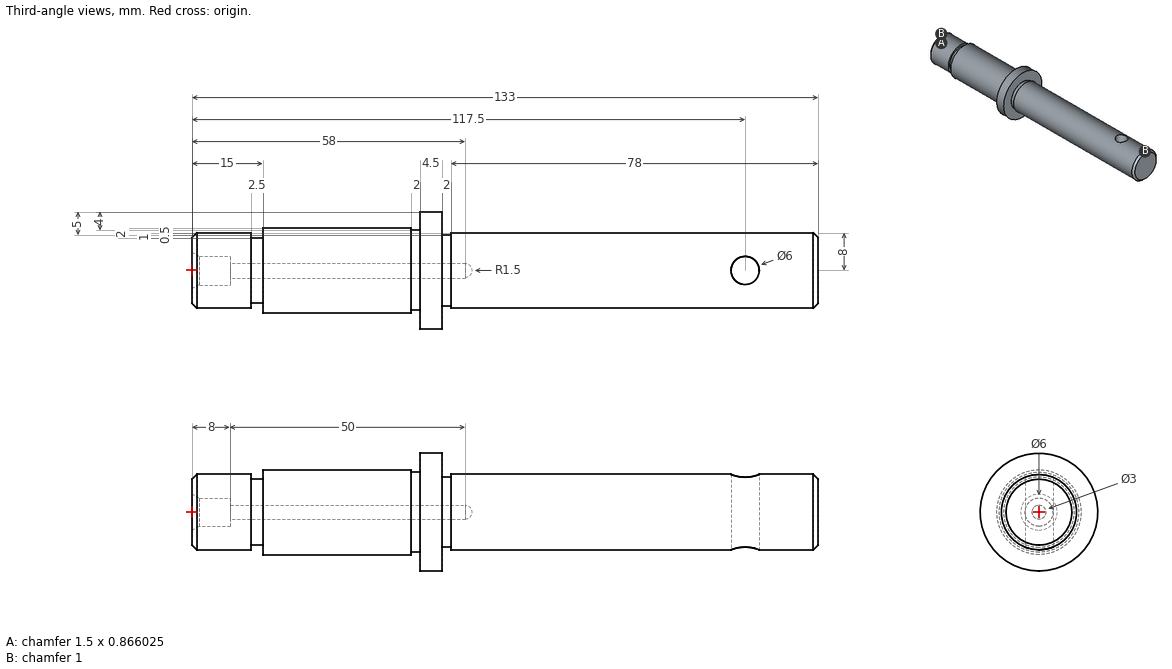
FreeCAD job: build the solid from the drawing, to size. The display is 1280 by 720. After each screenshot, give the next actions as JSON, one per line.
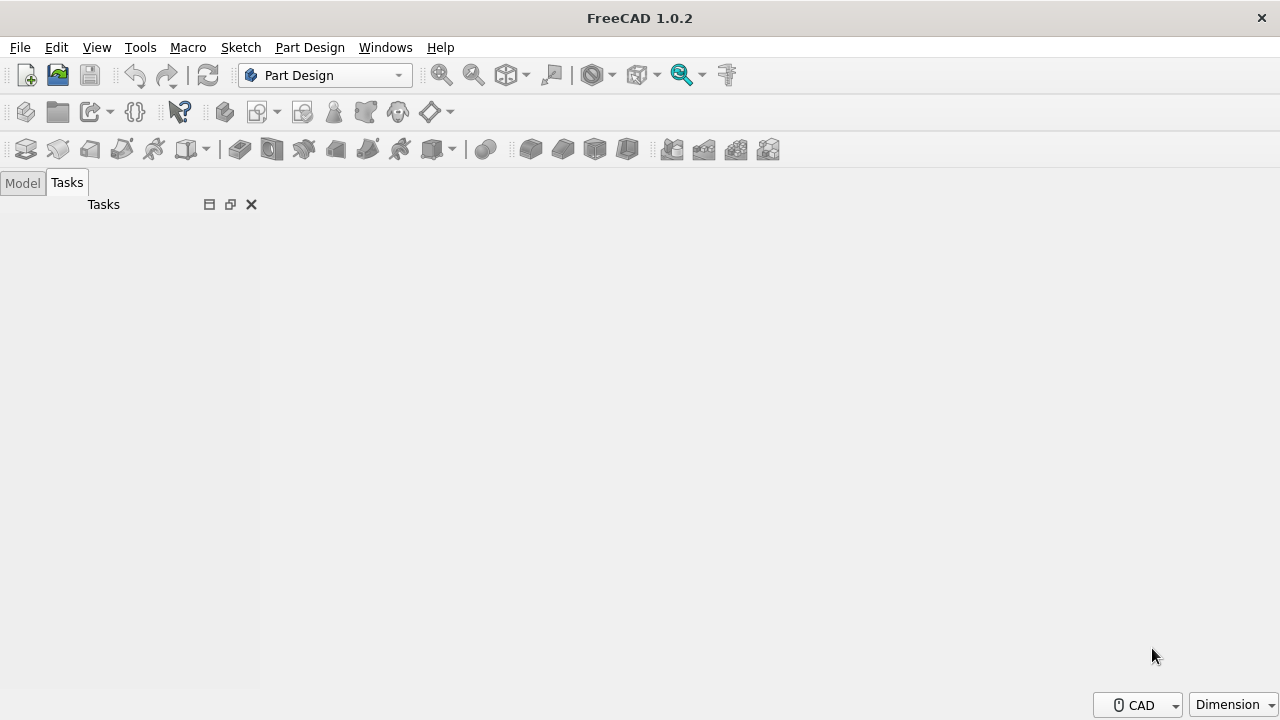
{"action": "left_click", "coordinate": [26, 76]}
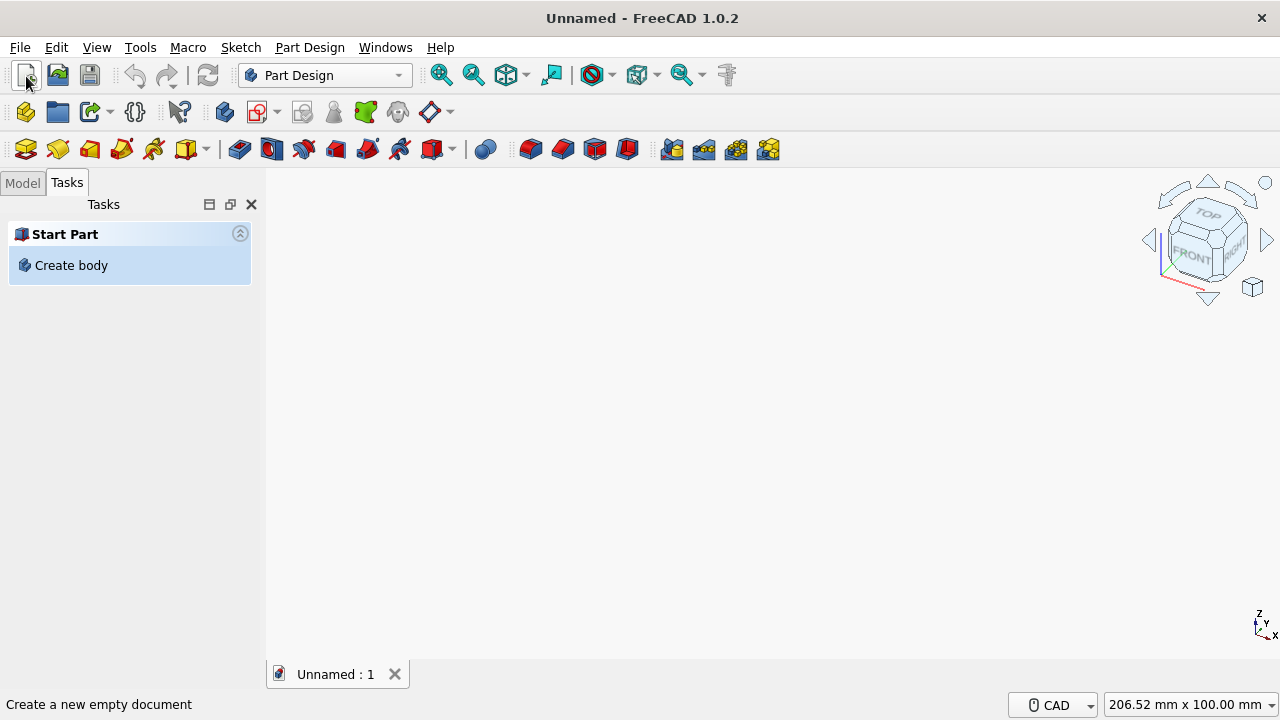
{"action": "left_click", "coordinate": [258, 112]}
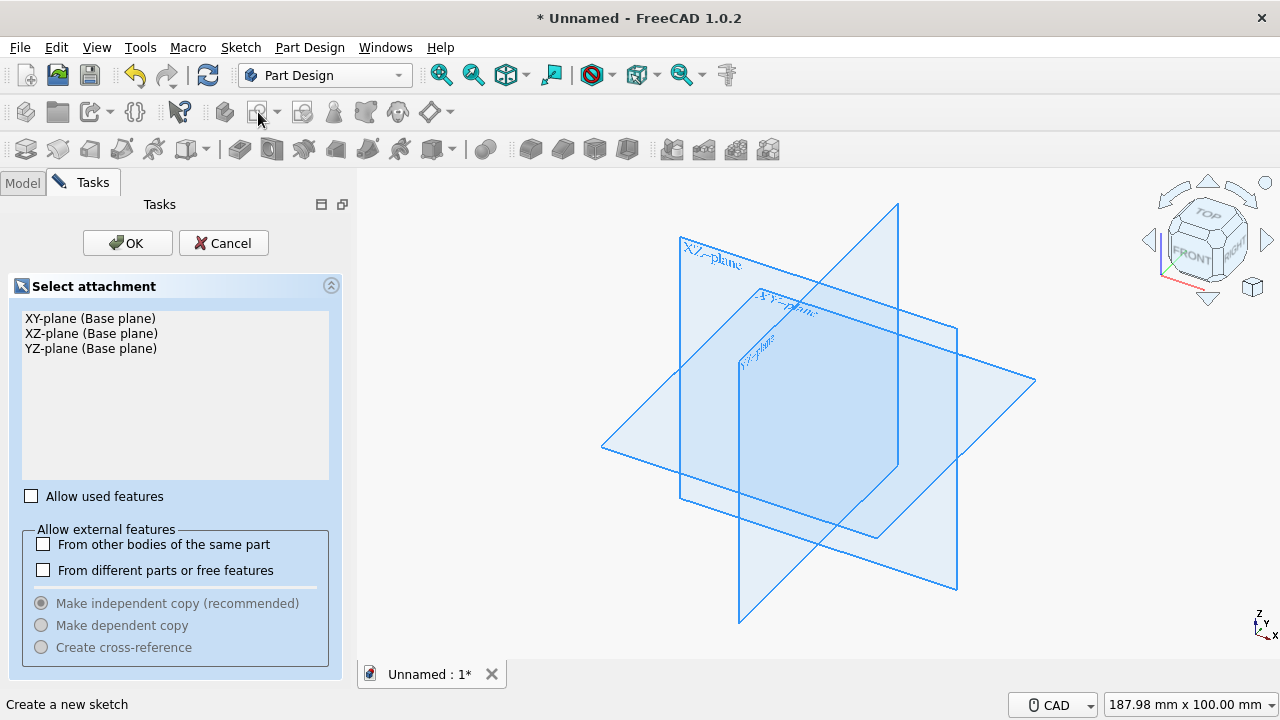
{"action": "left_click", "coordinate": [82, 318]}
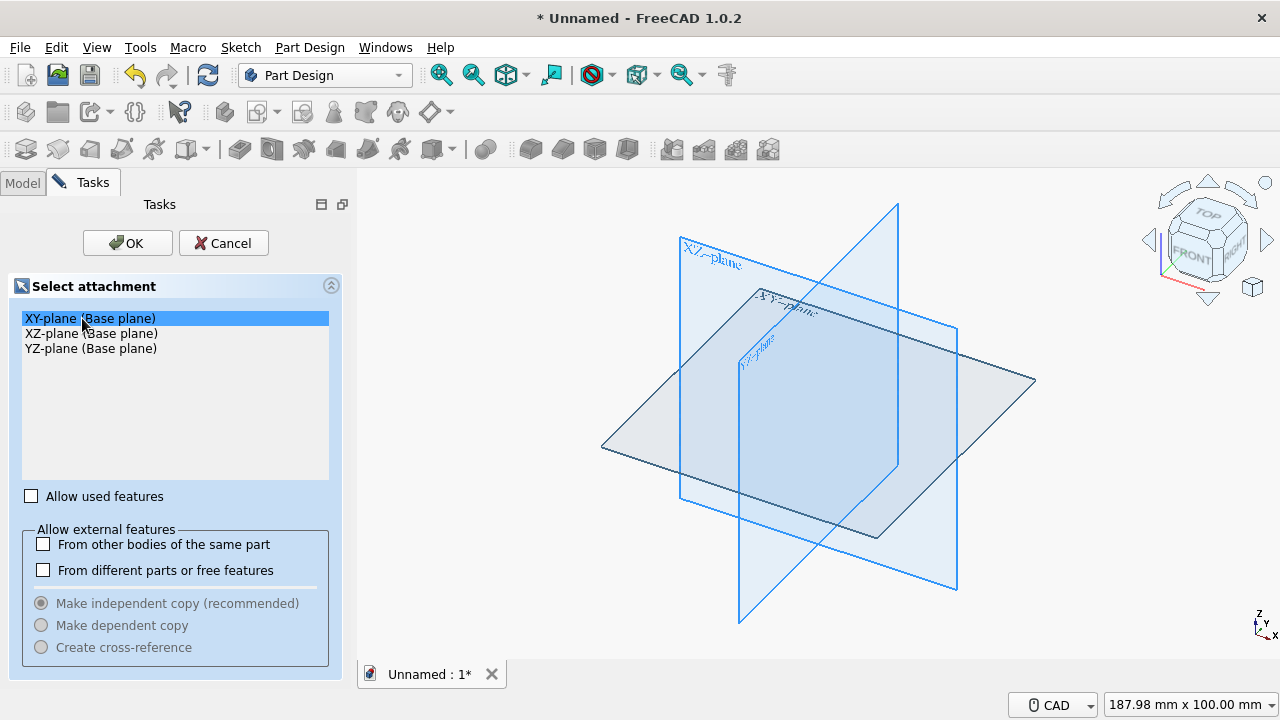
{"action": "left_click", "coordinate": [128, 243]}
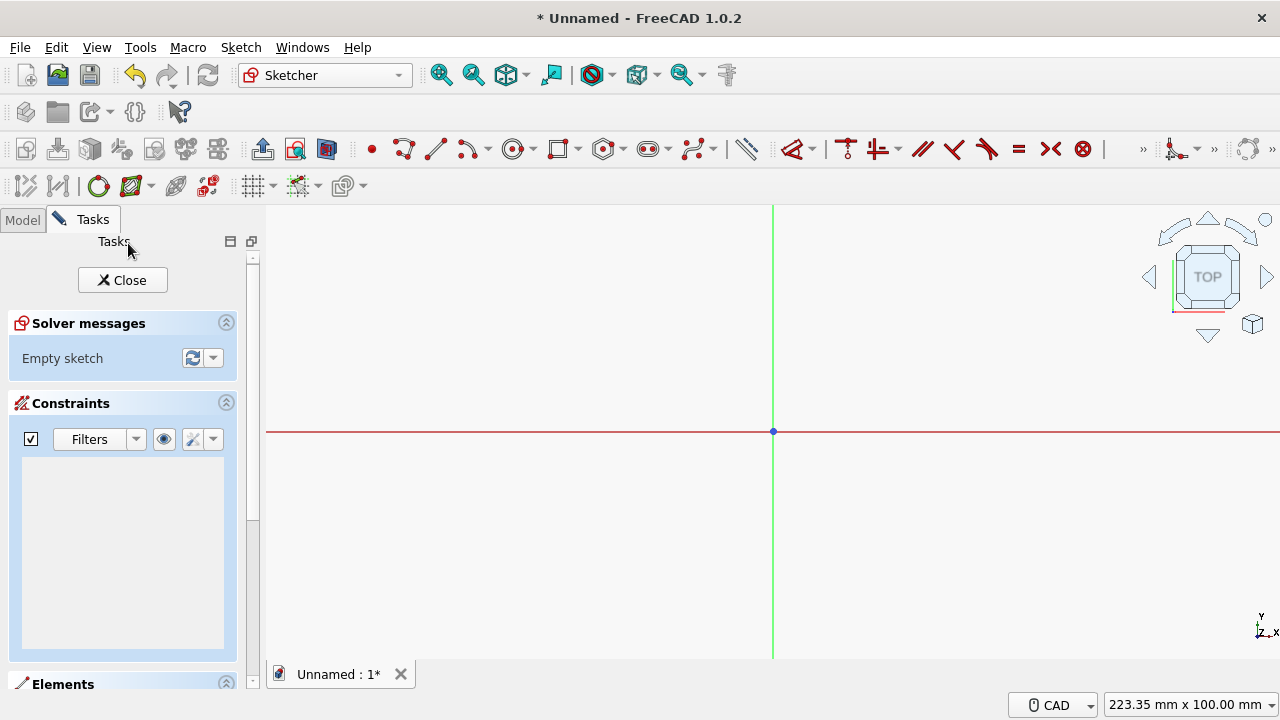
{"action": "scroll", "coordinate": [294, 490], "scroll_direction": "down", "scroll_amount": 2}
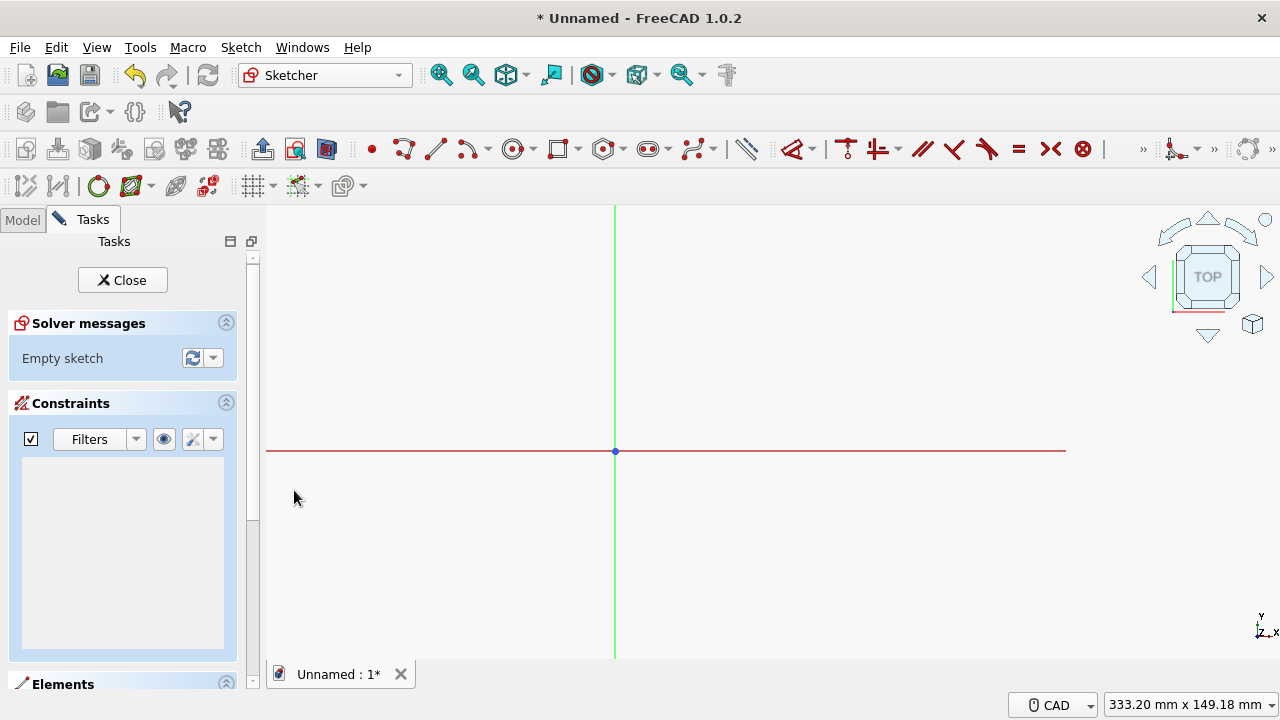
{"action": "scroll", "coordinate": [1047, 433], "scroll_direction": "up", "scroll_amount": 2}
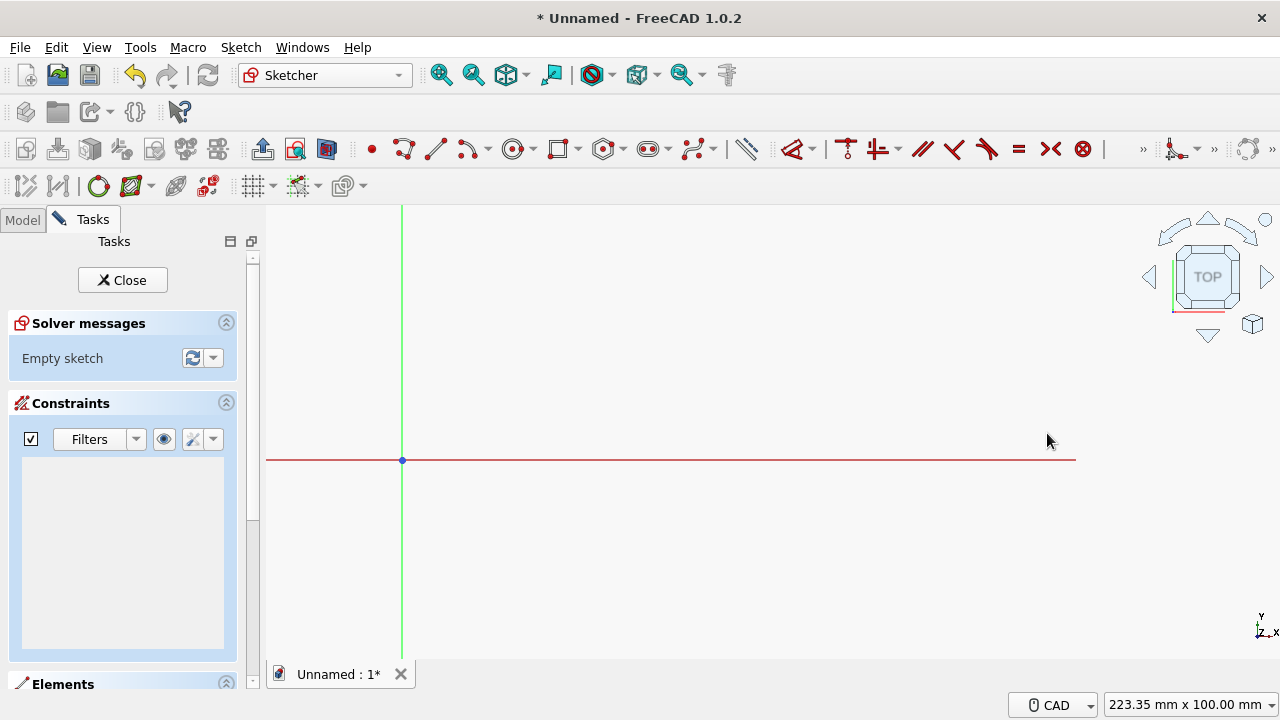
{"action": "key", "text": "g m"}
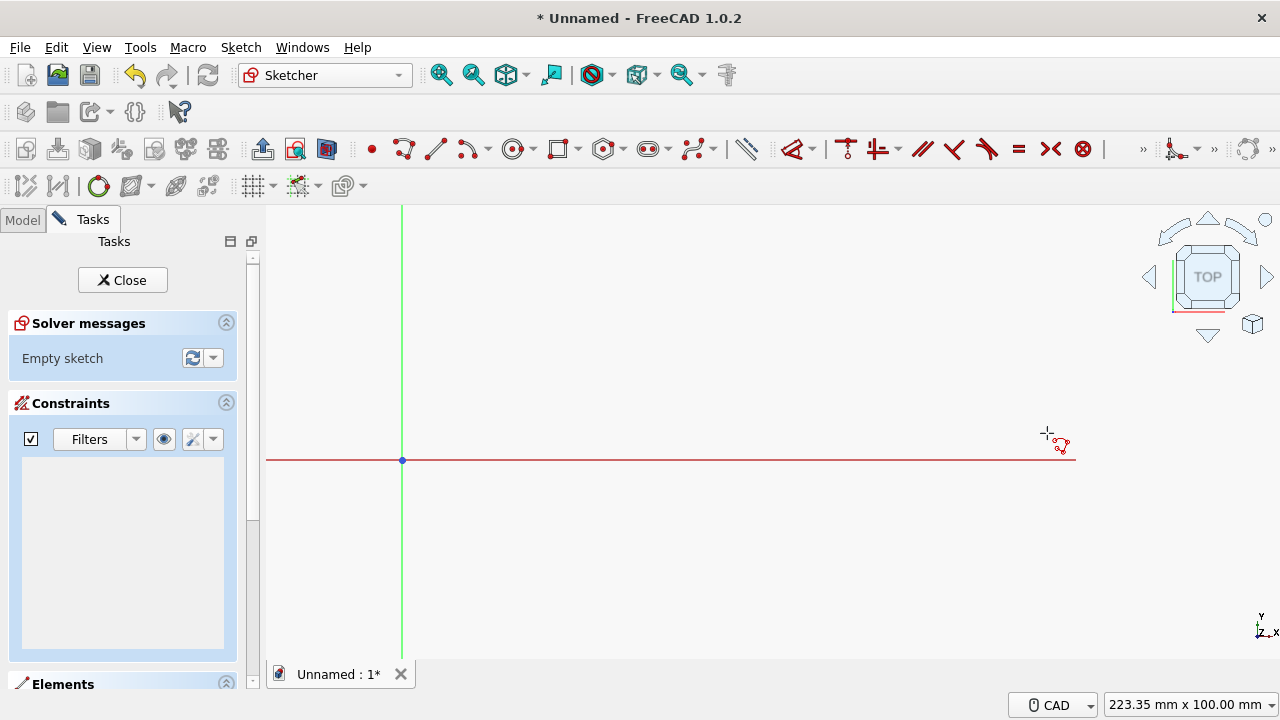
{"action": "left_click", "coordinate": [402, 460]}
{"action": "left_click", "coordinate": [1006, 451]}
{"action": "left_click", "coordinate": [1006, 424]}
{"action": "left_click", "coordinate": [652, 424]}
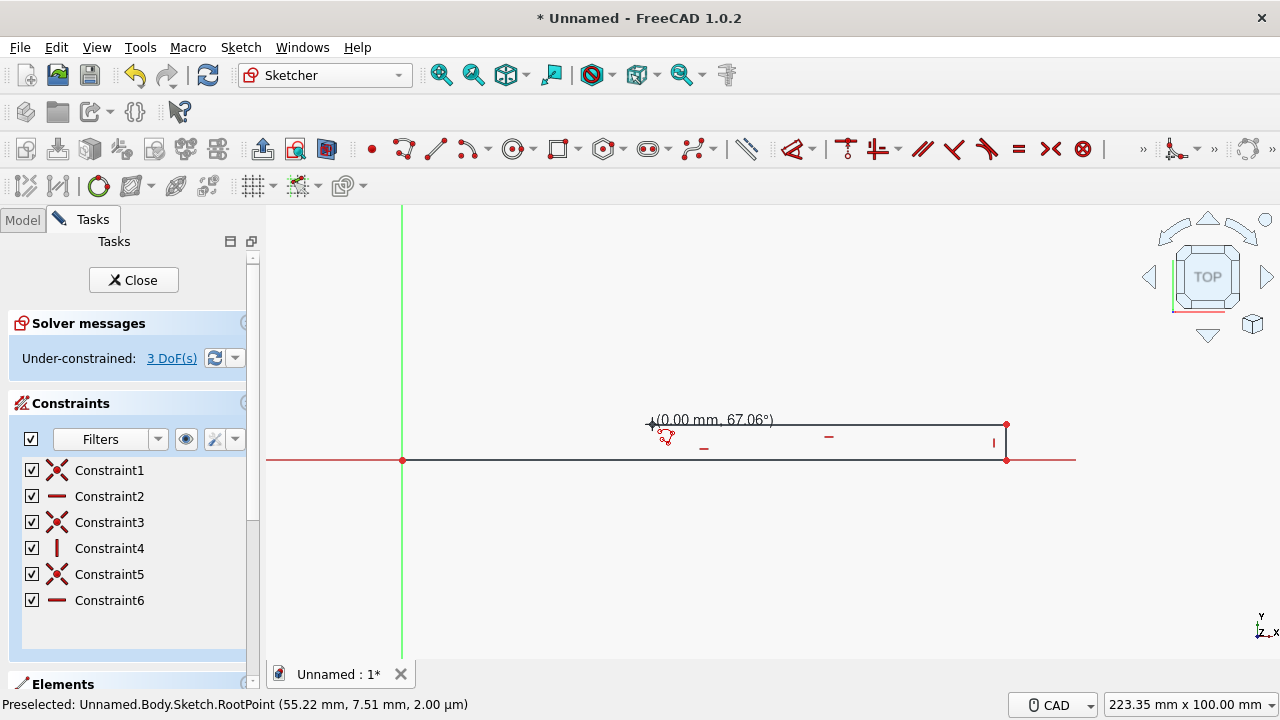
{"action": "scroll", "coordinate": [652, 426], "scroll_direction": "up", "scroll_amount": 10}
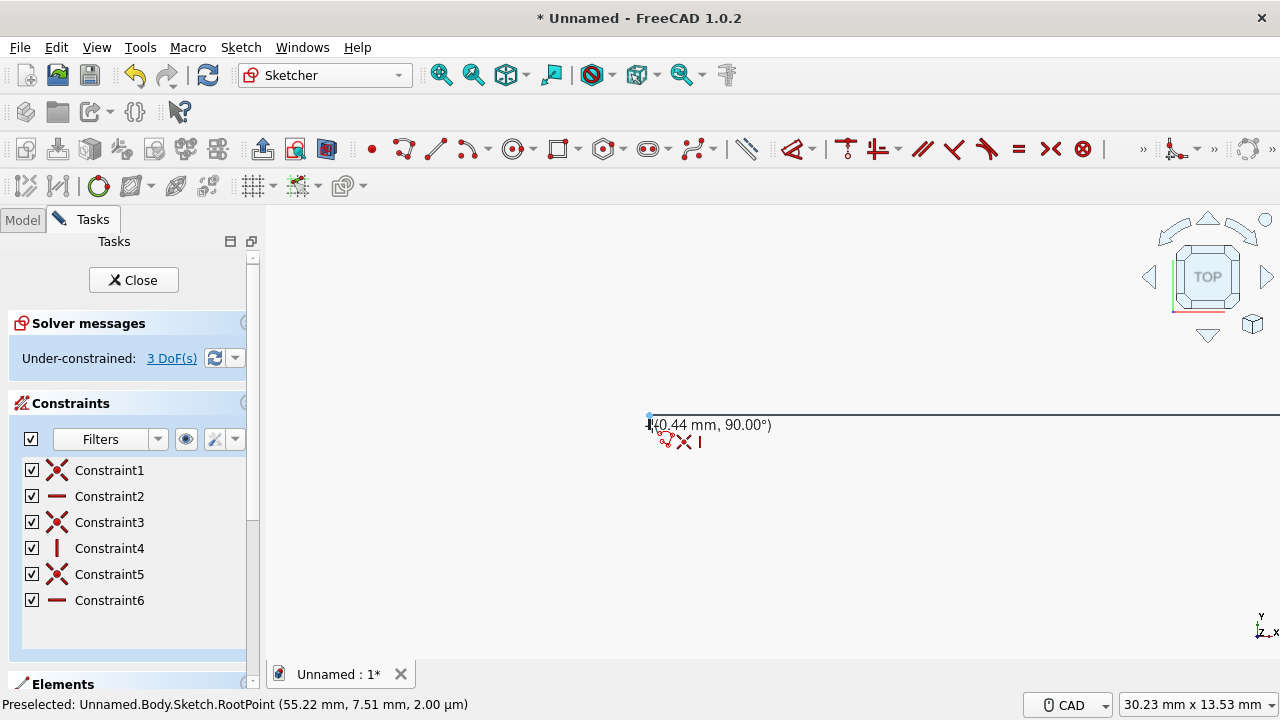
{"action": "left_click", "coordinate": [650, 423]}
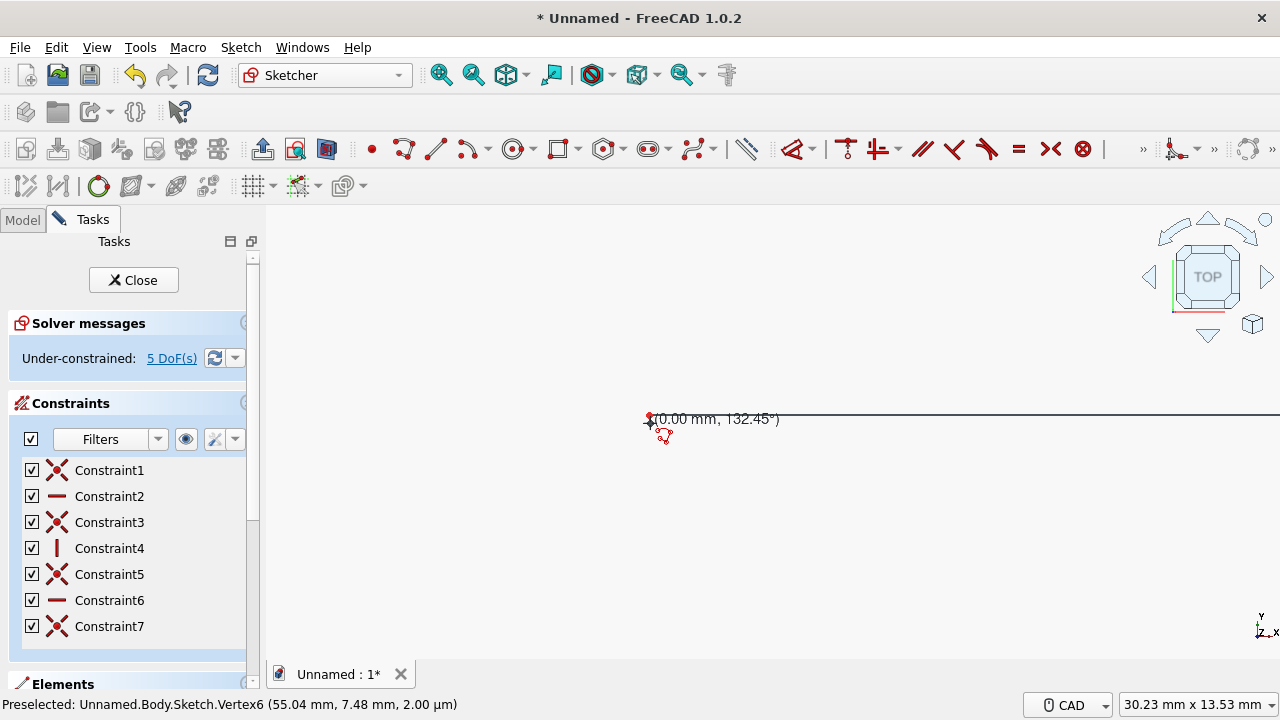
{"action": "scroll", "coordinate": [653, 427], "scroll_direction": "down", "scroll_amount": 10}